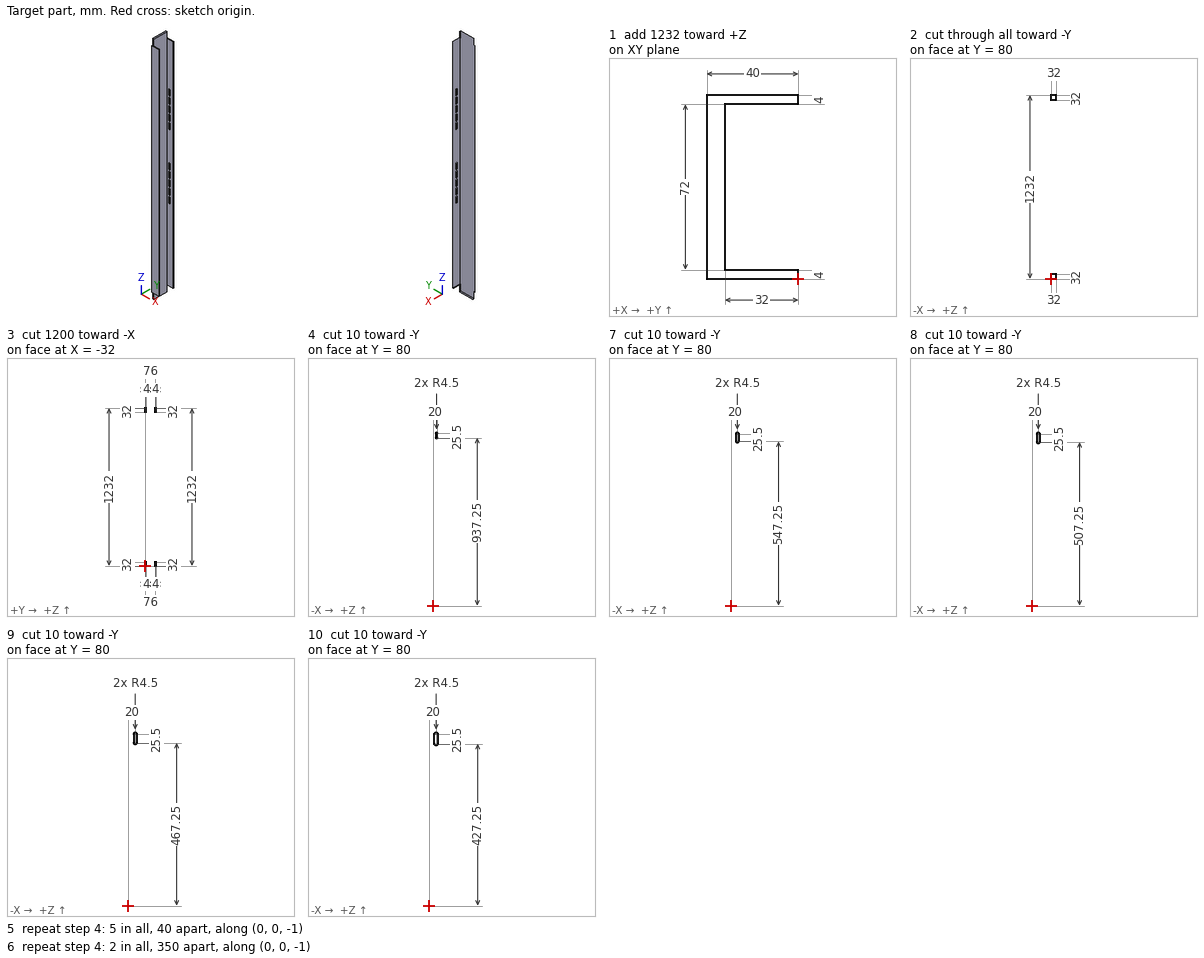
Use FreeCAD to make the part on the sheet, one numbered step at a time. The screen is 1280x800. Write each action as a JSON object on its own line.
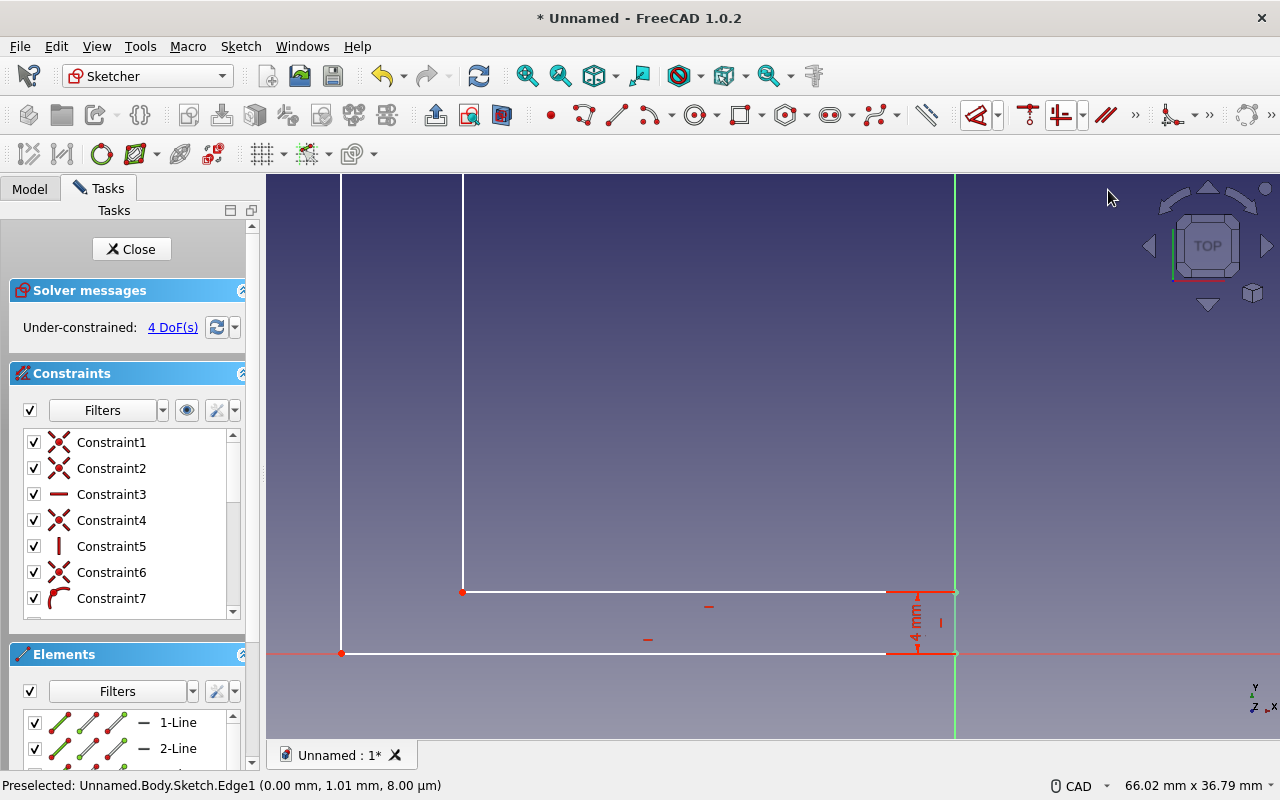
{"action": "scroll", "coordinate": [729, 636], "scroll_direction": "down", "scroll_amount": 6}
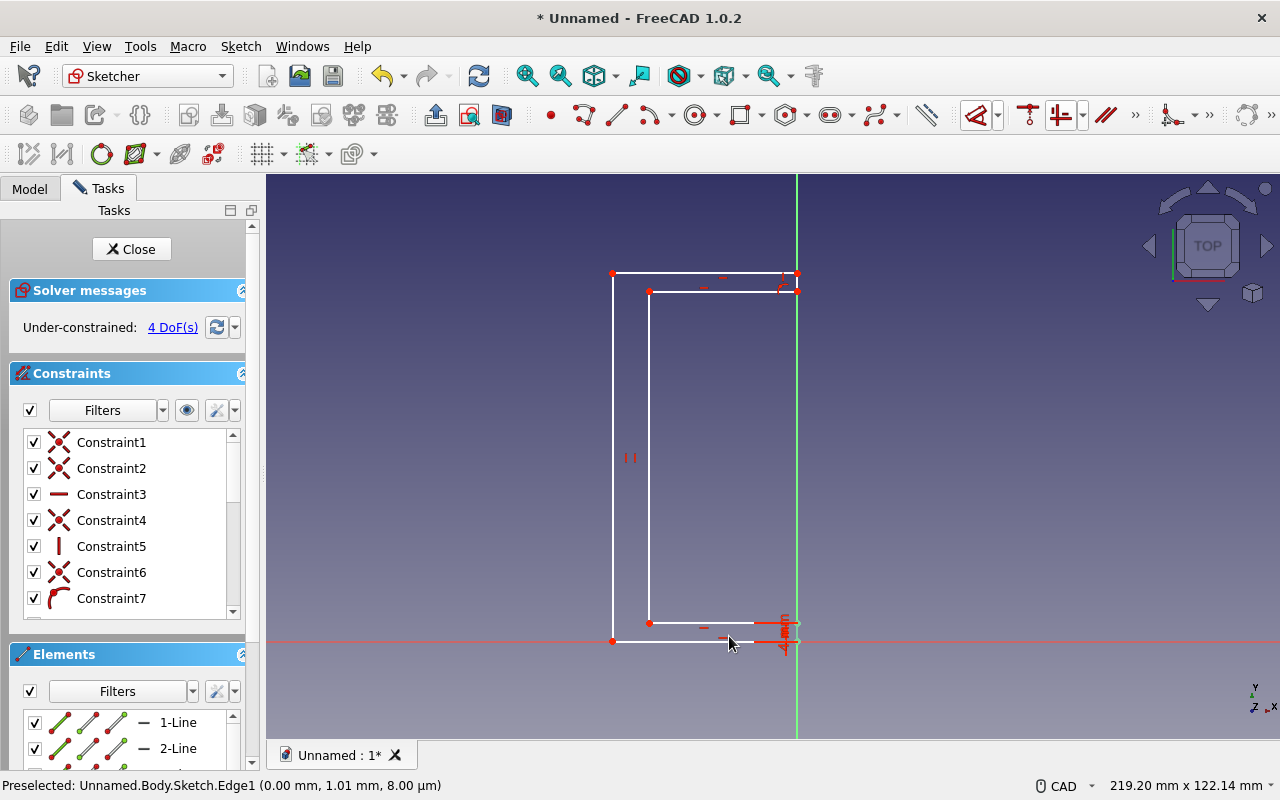
{"action": "scroll", "coordinate": [797, 286], "scroll_direction": "up", "scroll_amount": 5}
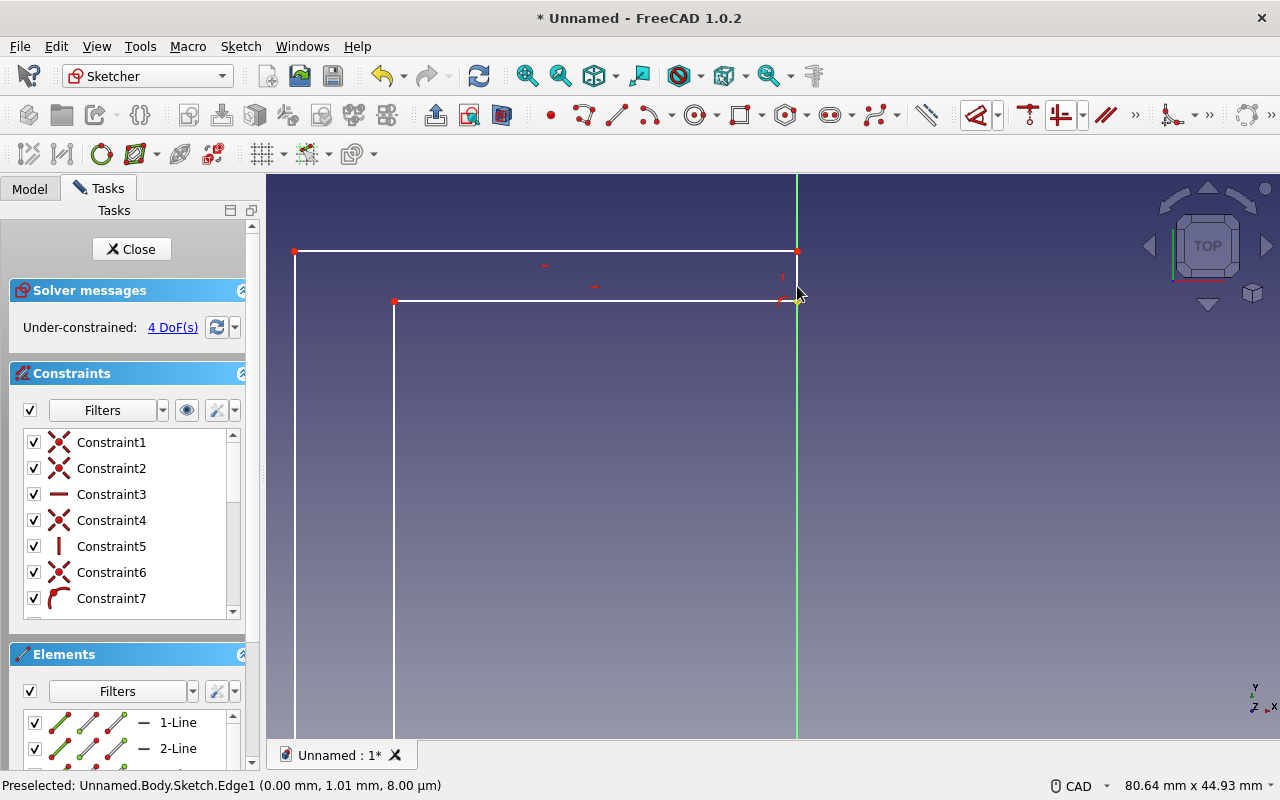
{"action": "left_click", "coordinate": [797, 286]}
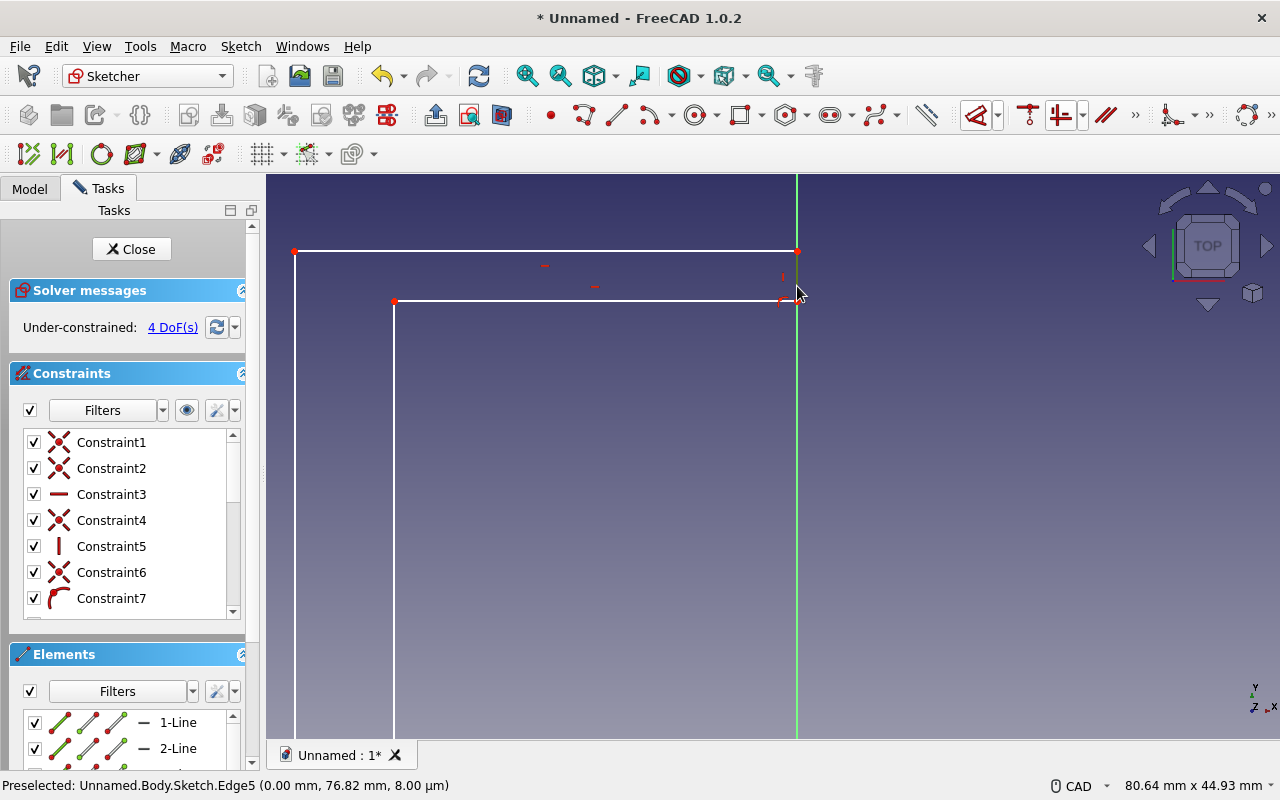
{"action": "key", "text": "i"}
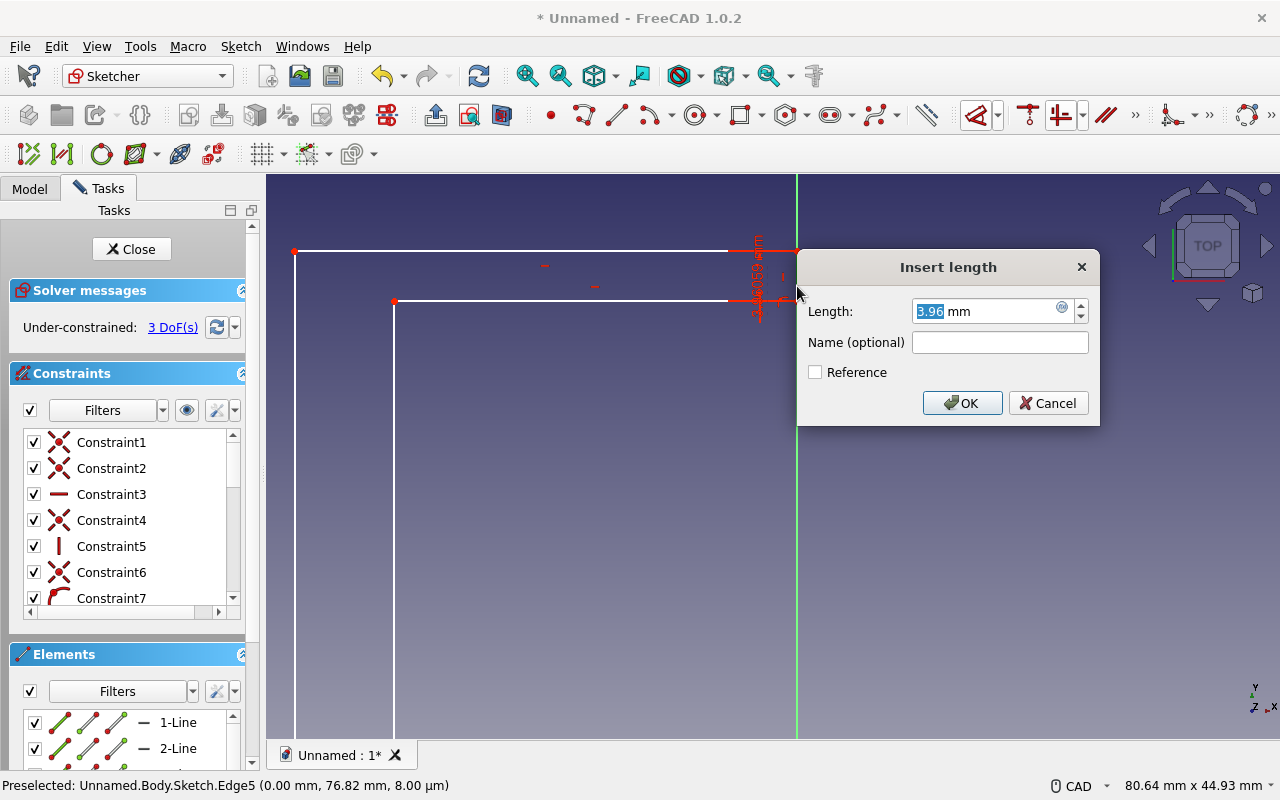
{"action": "type", "text": "4"}
{"action": "key", "text": "Return"}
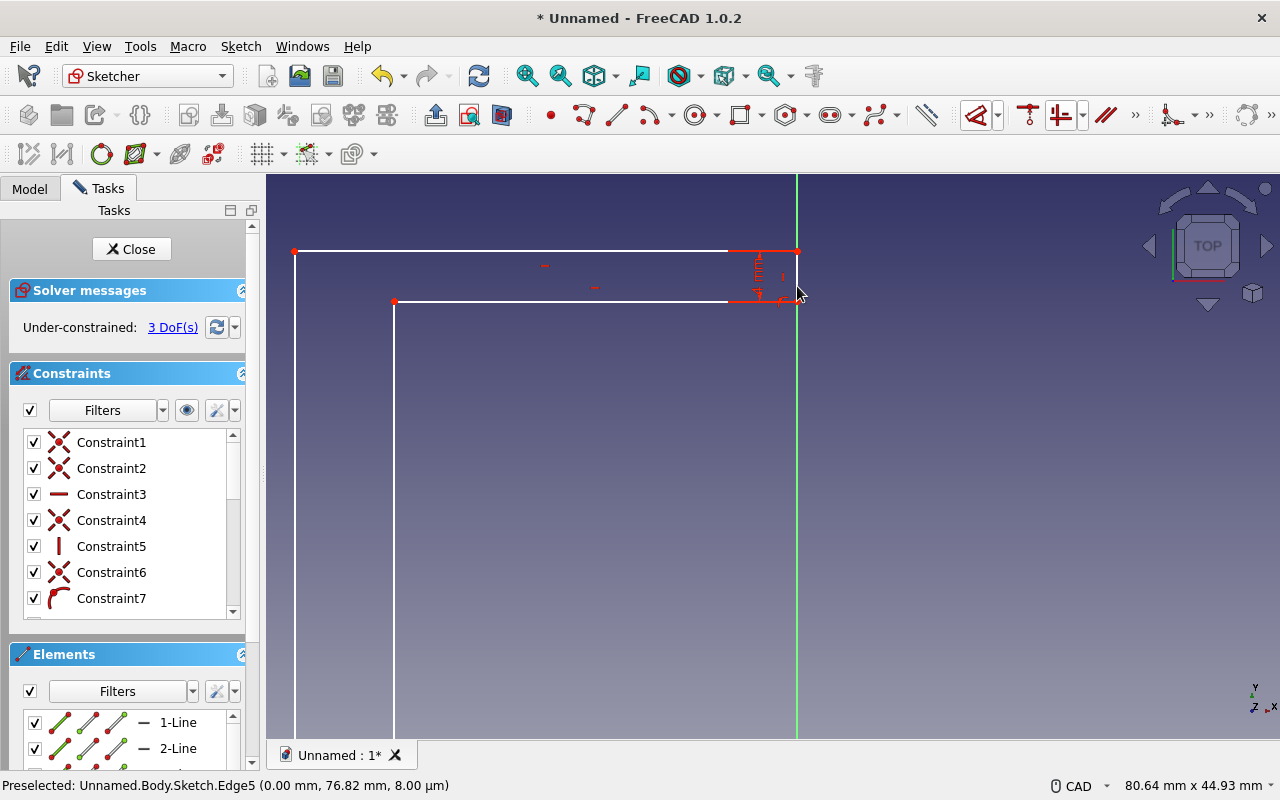
{"action": "scroll", "coordinate": [797, 286], "scroll_direction": "down", "scroll_amount": 5}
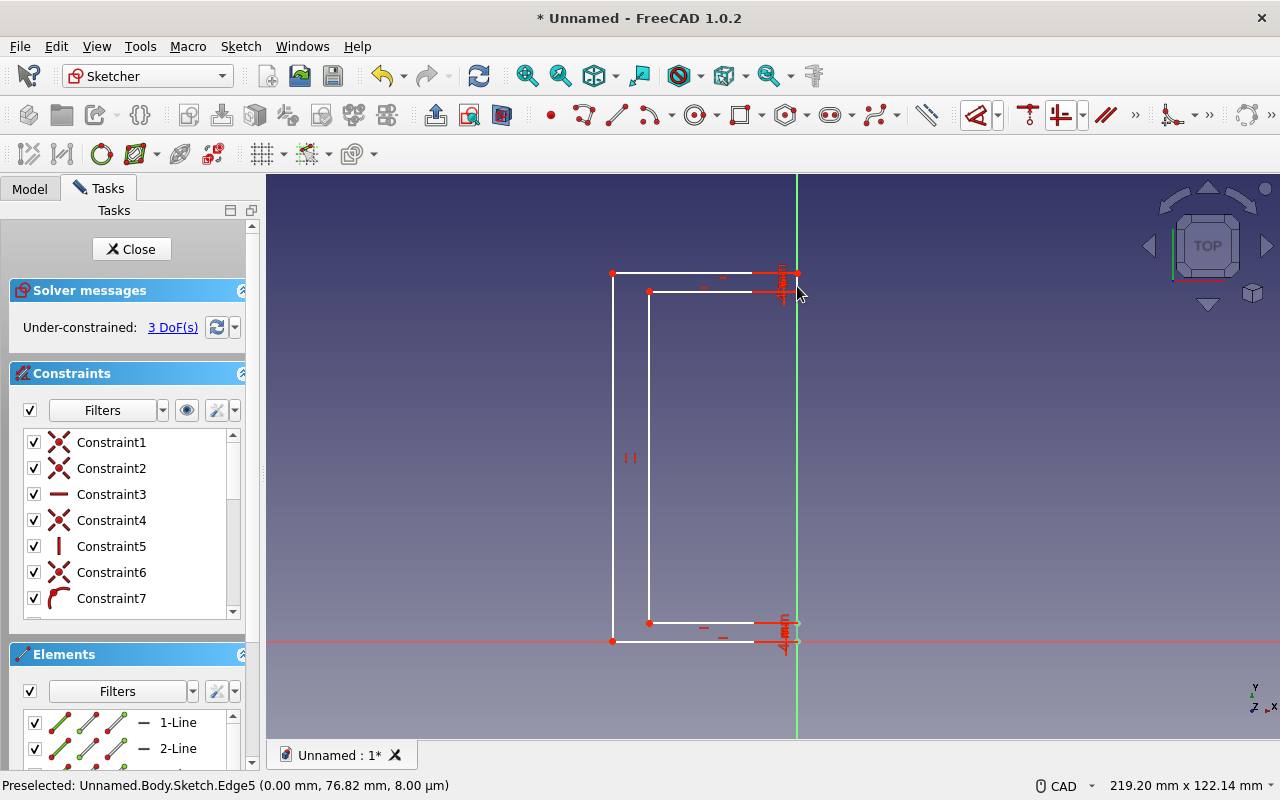
{"action": "left_click", "coordinate": [753, 623]}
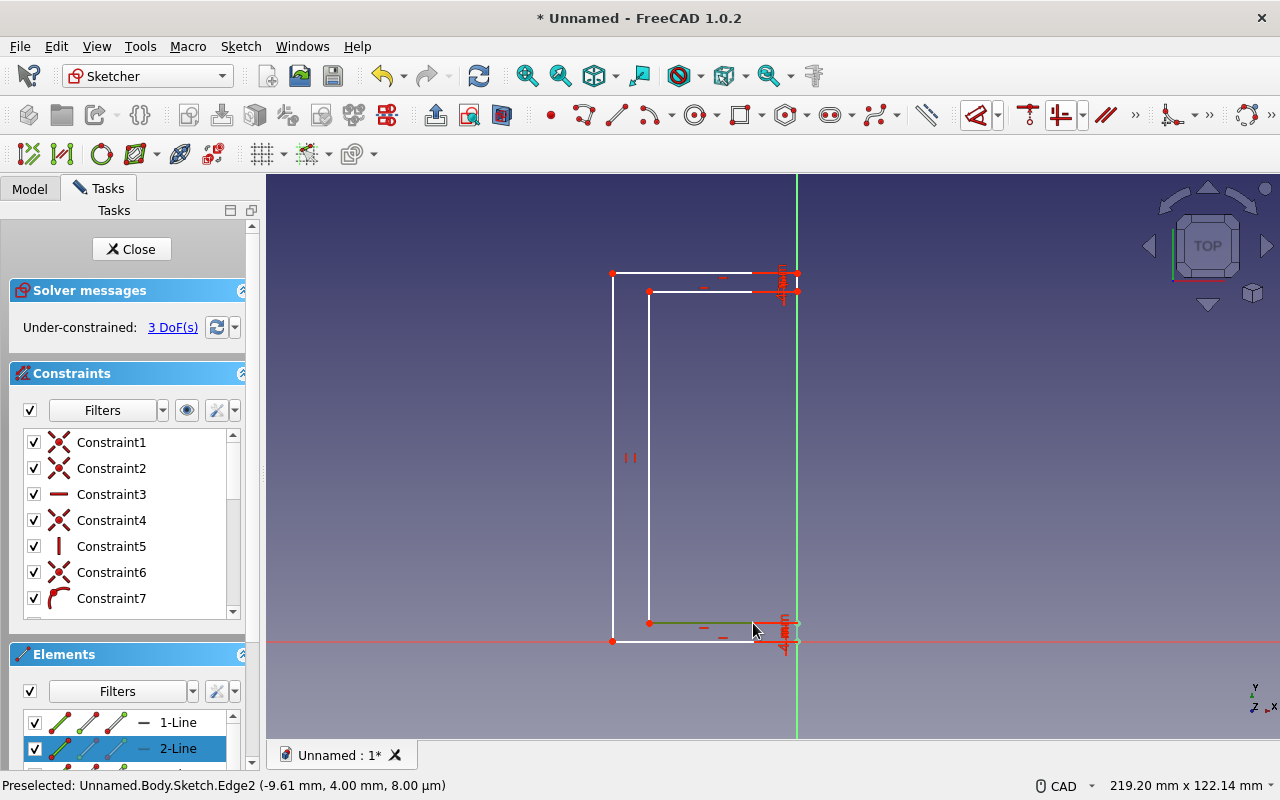
{"action": "key", "text": "l"}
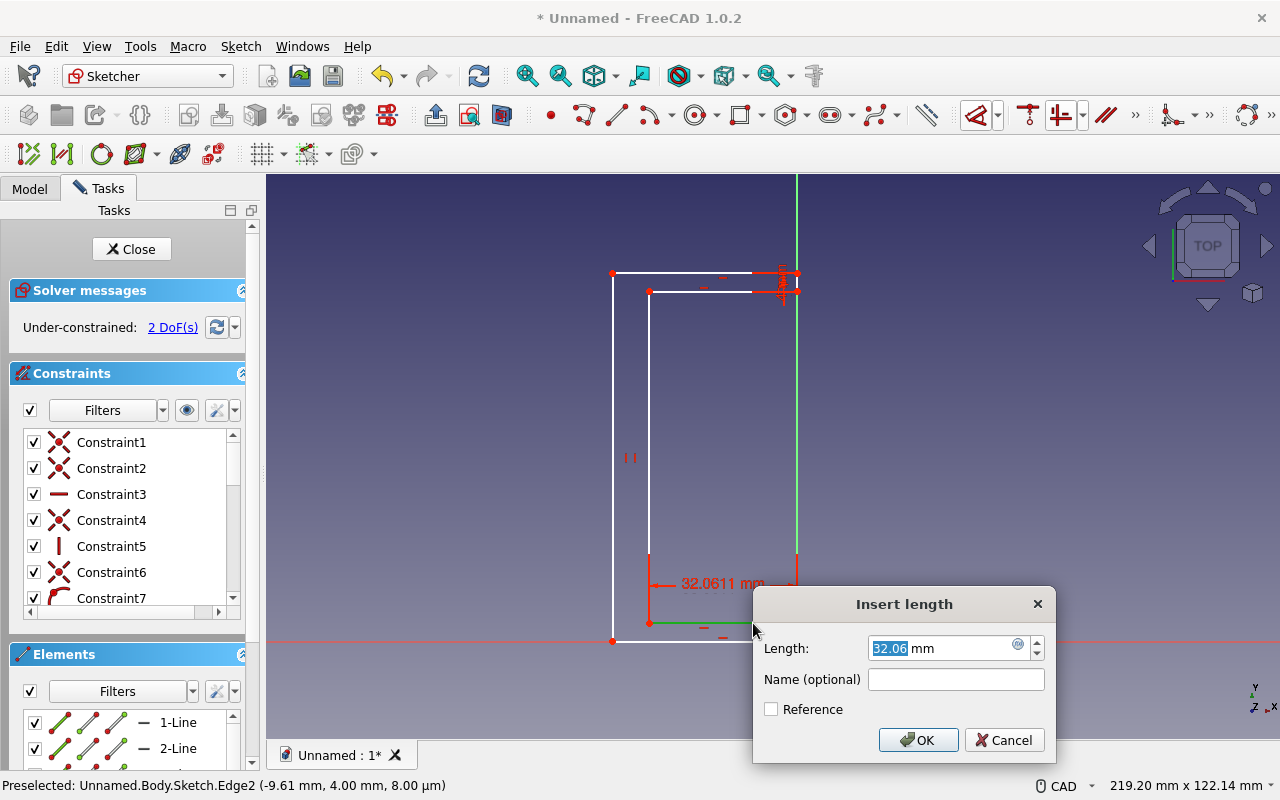
{"action": "type", "text": "32"}
{"action": "key", "text": "Return"}